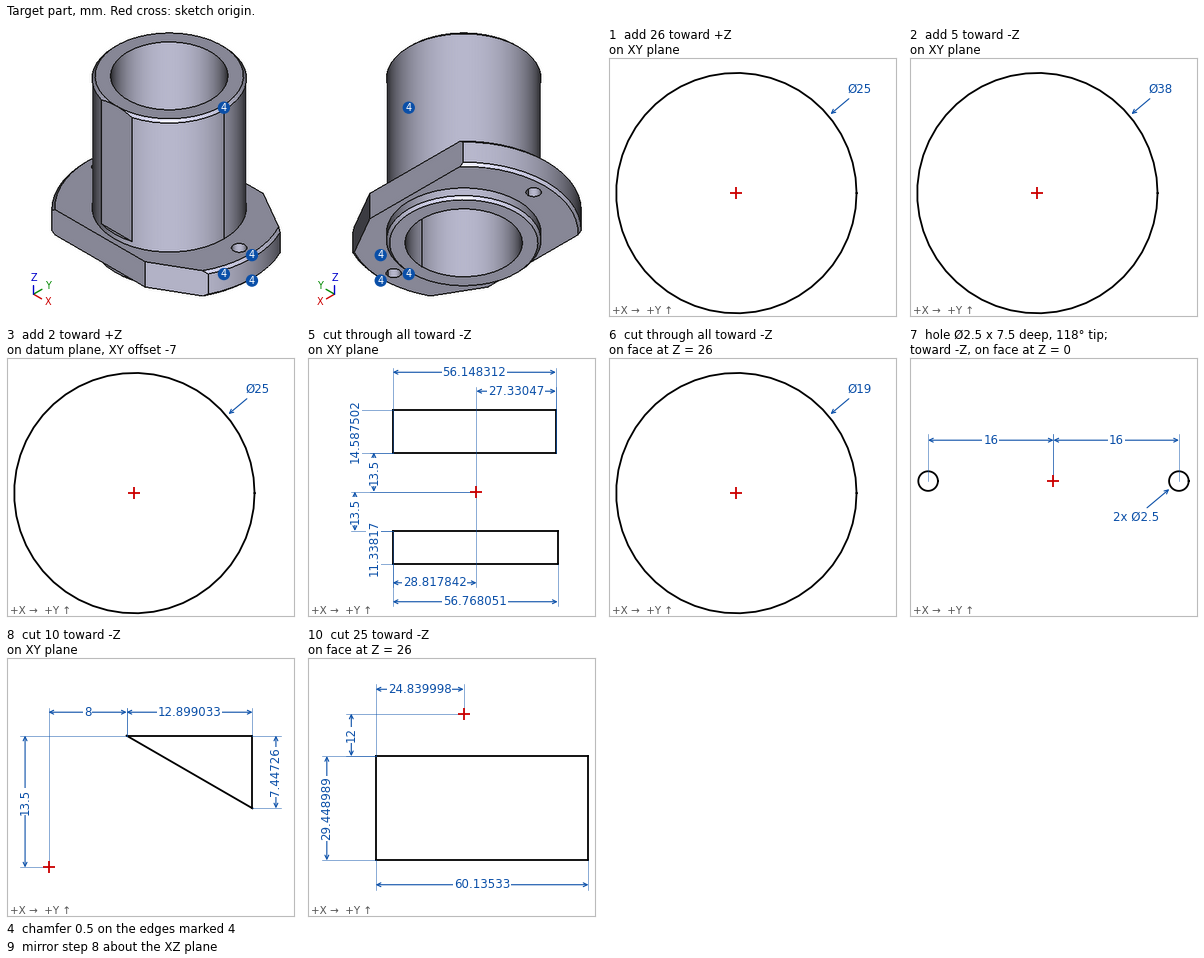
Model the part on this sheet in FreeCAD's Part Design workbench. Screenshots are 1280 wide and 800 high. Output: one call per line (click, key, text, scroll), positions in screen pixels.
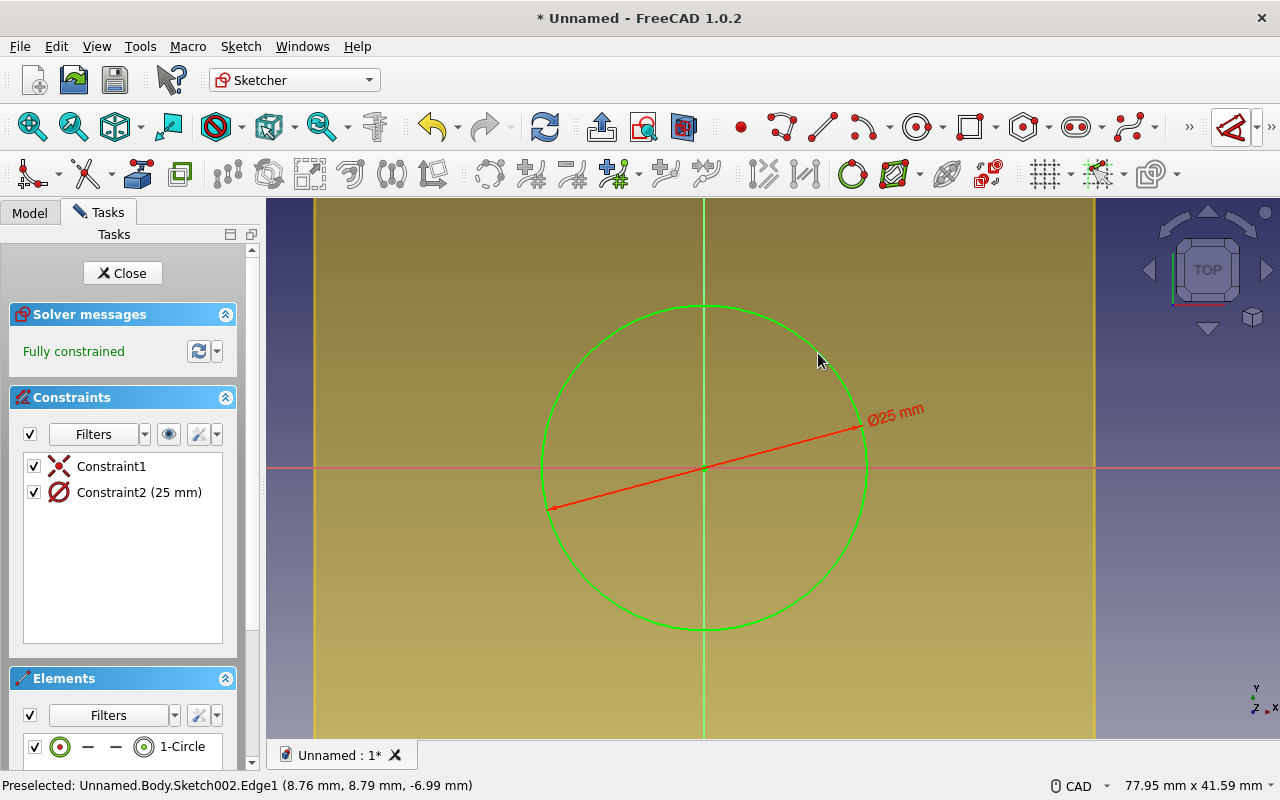
click(123, 273)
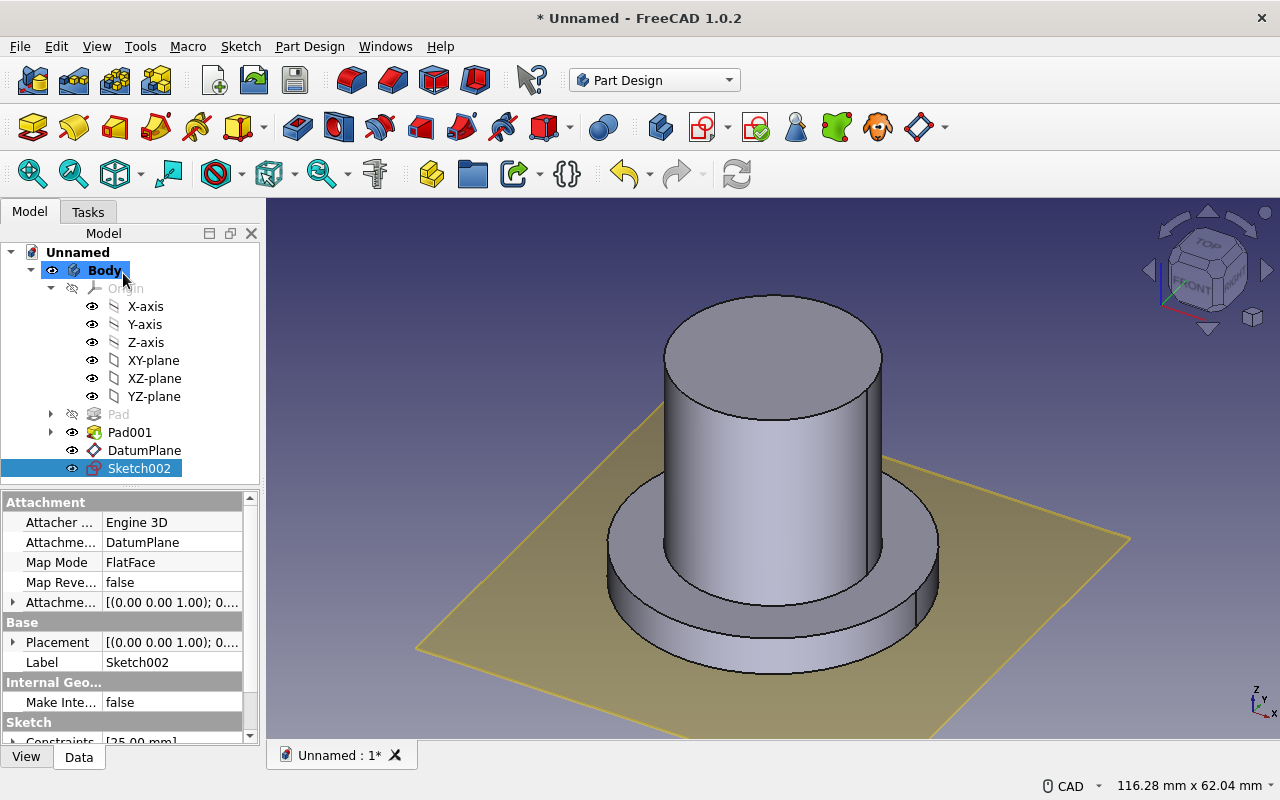
click(33, 128)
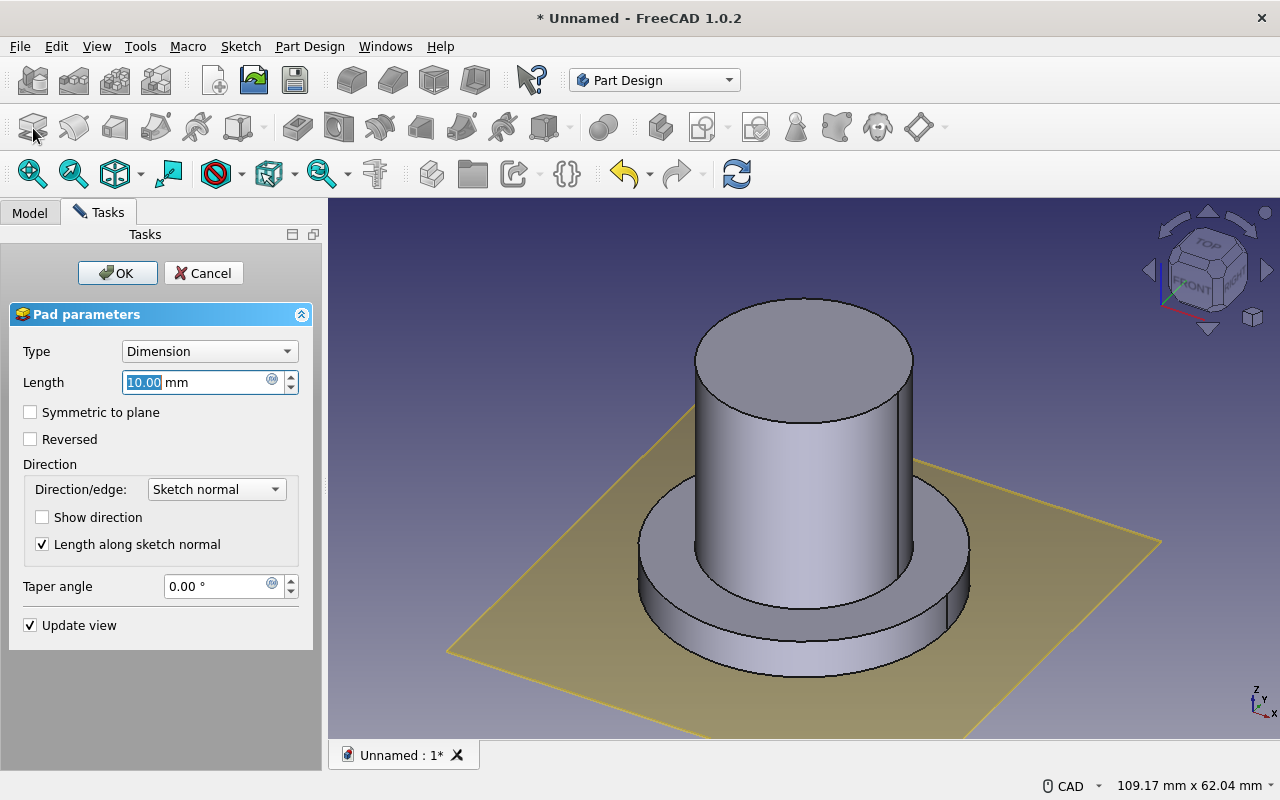
text(2)
key(Tab)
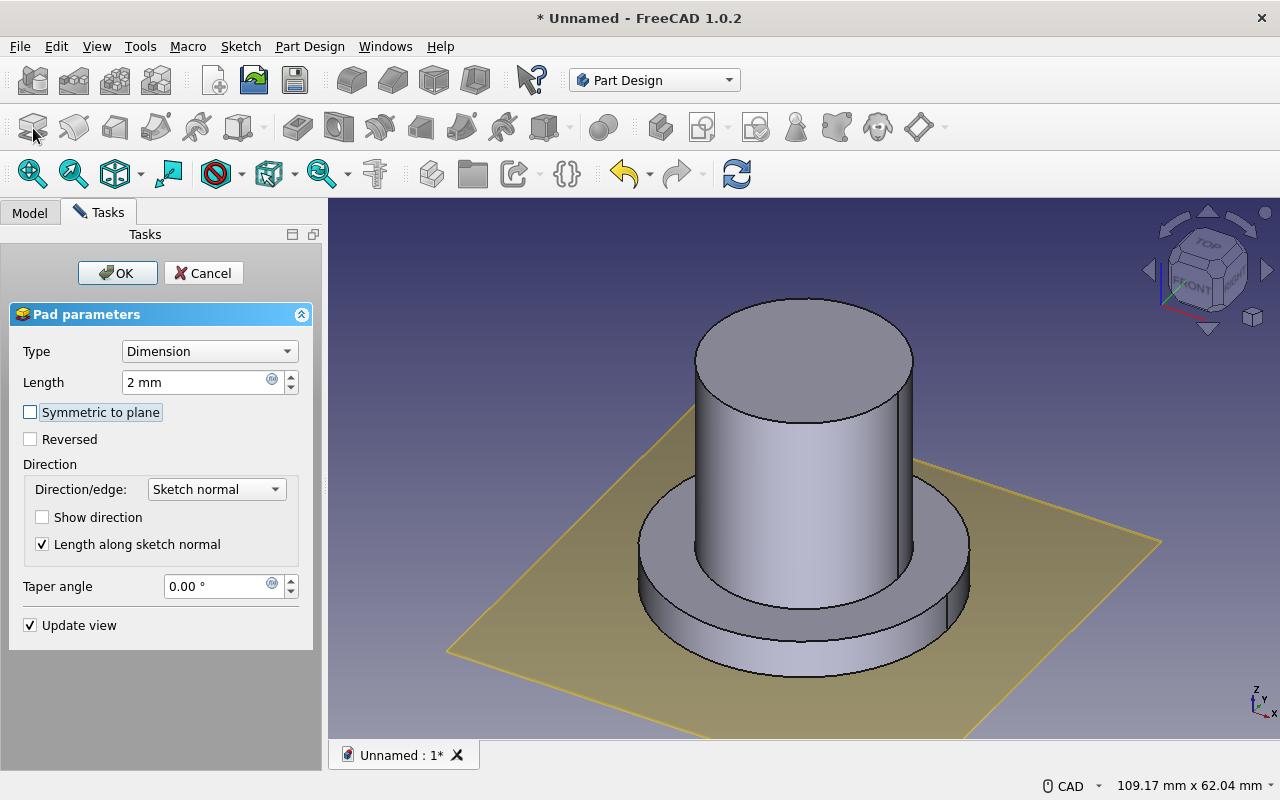
click(118, 273)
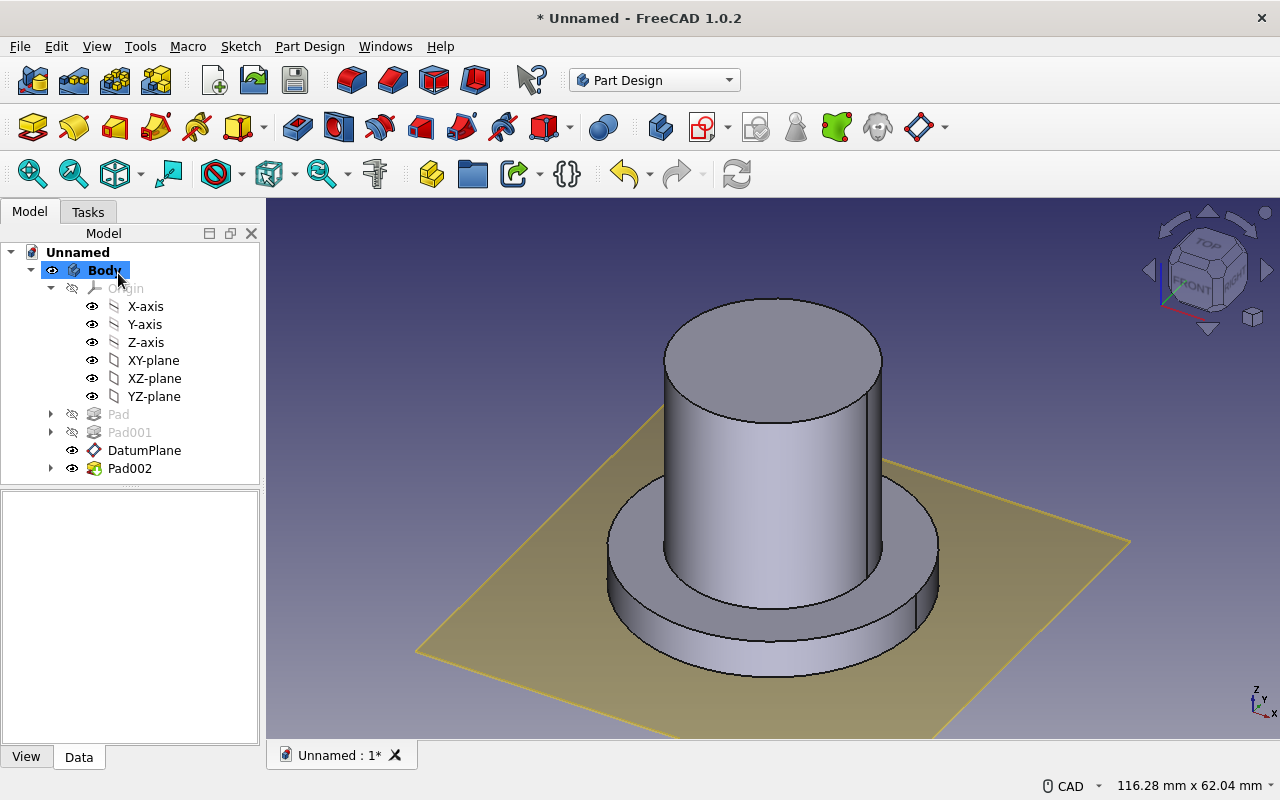
click(117, 450)
key(space)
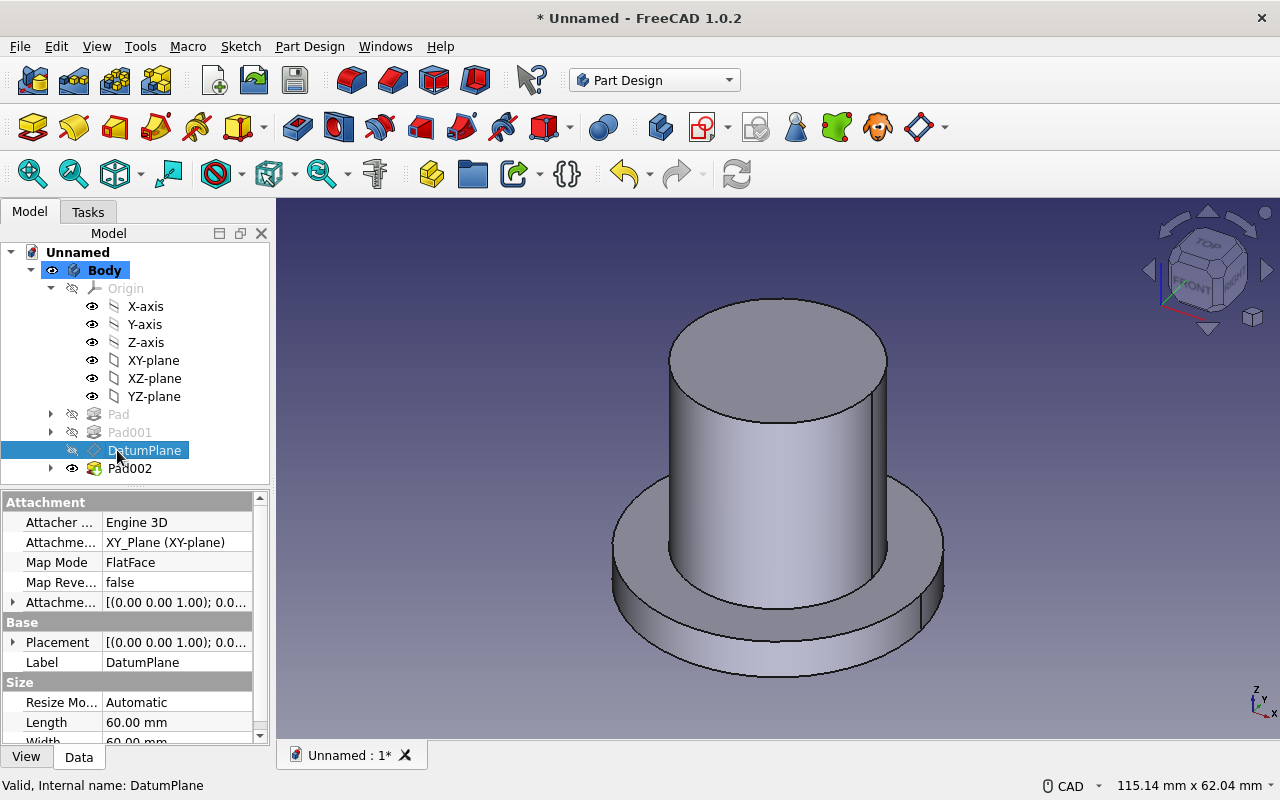
click(670, 366)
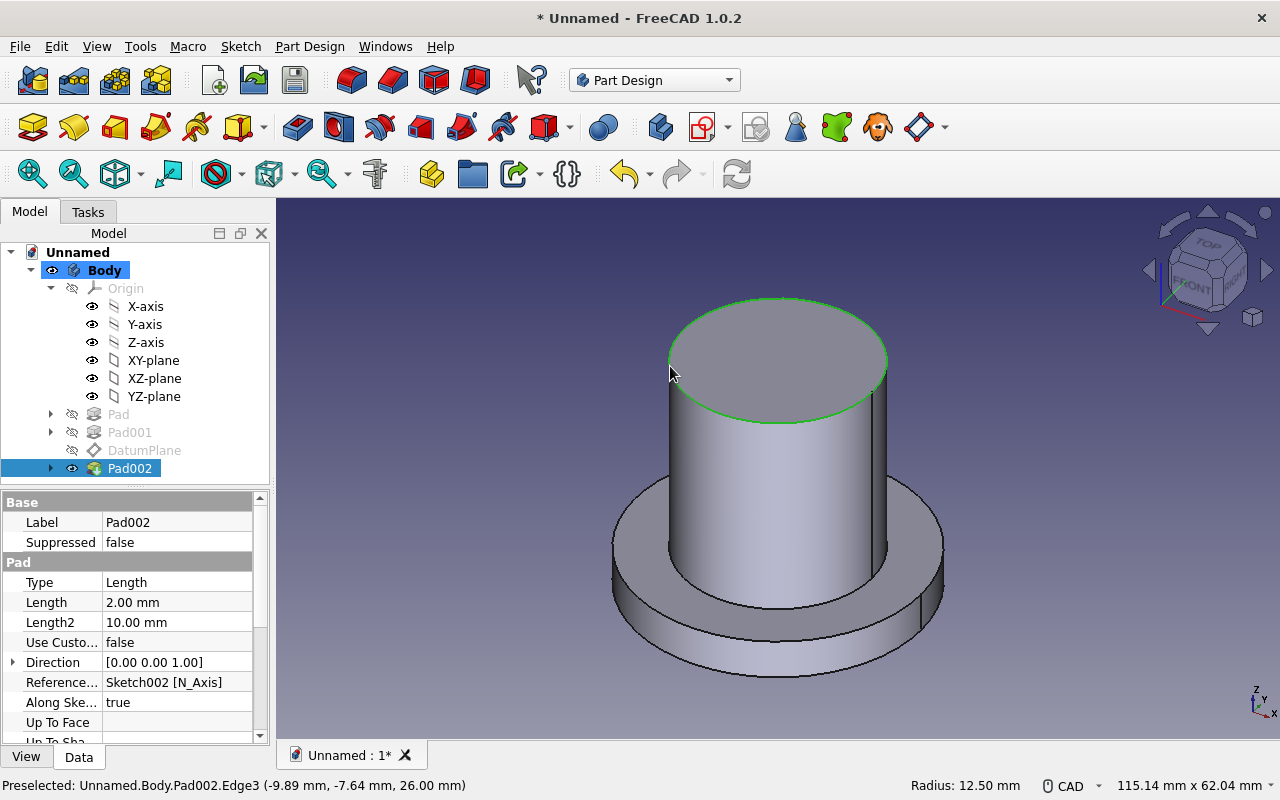
click(613, 556, ctrl)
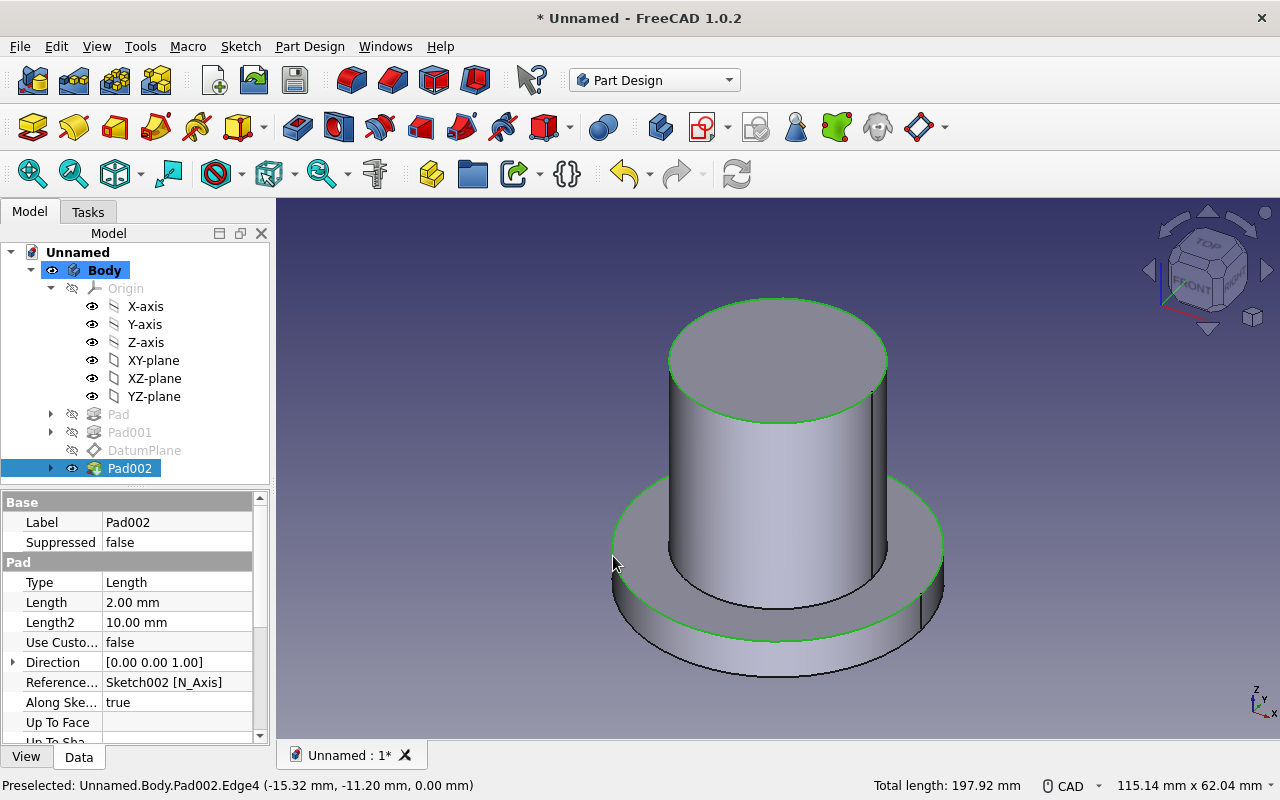
key(0)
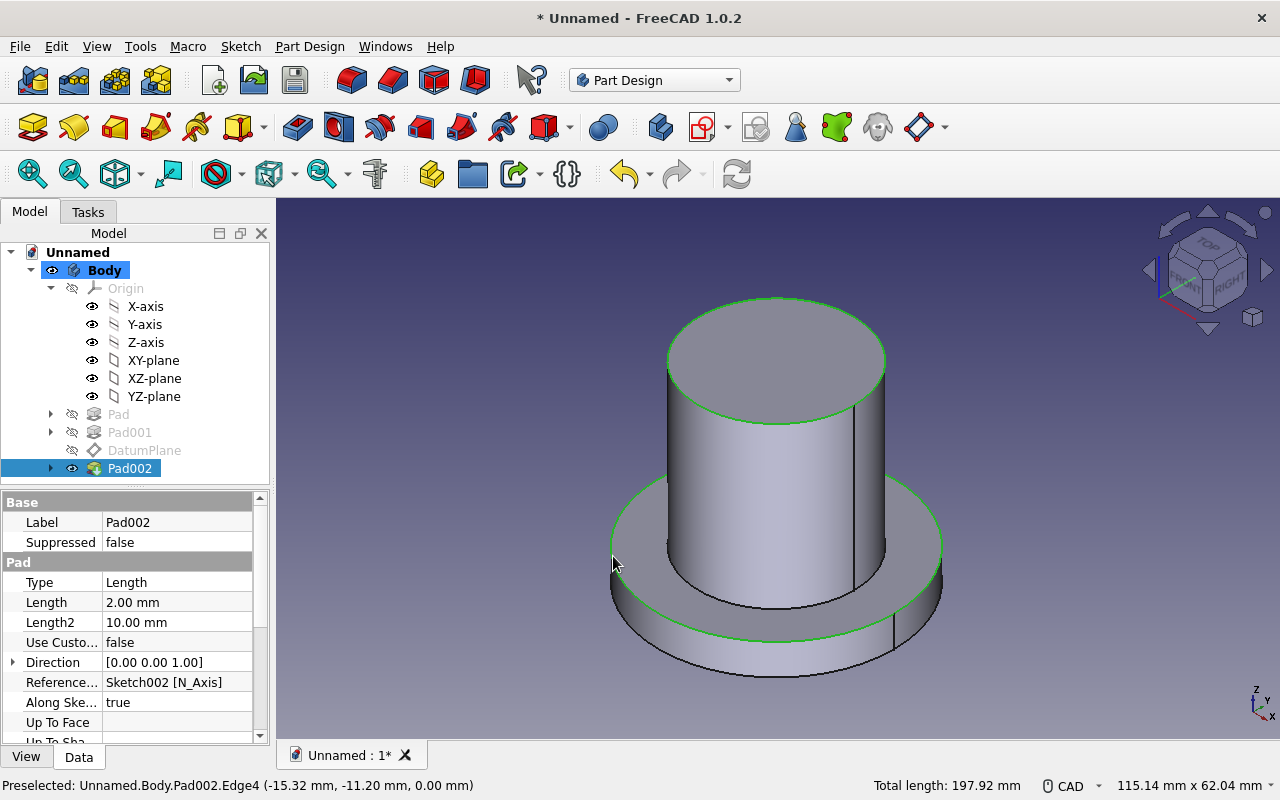
key(2)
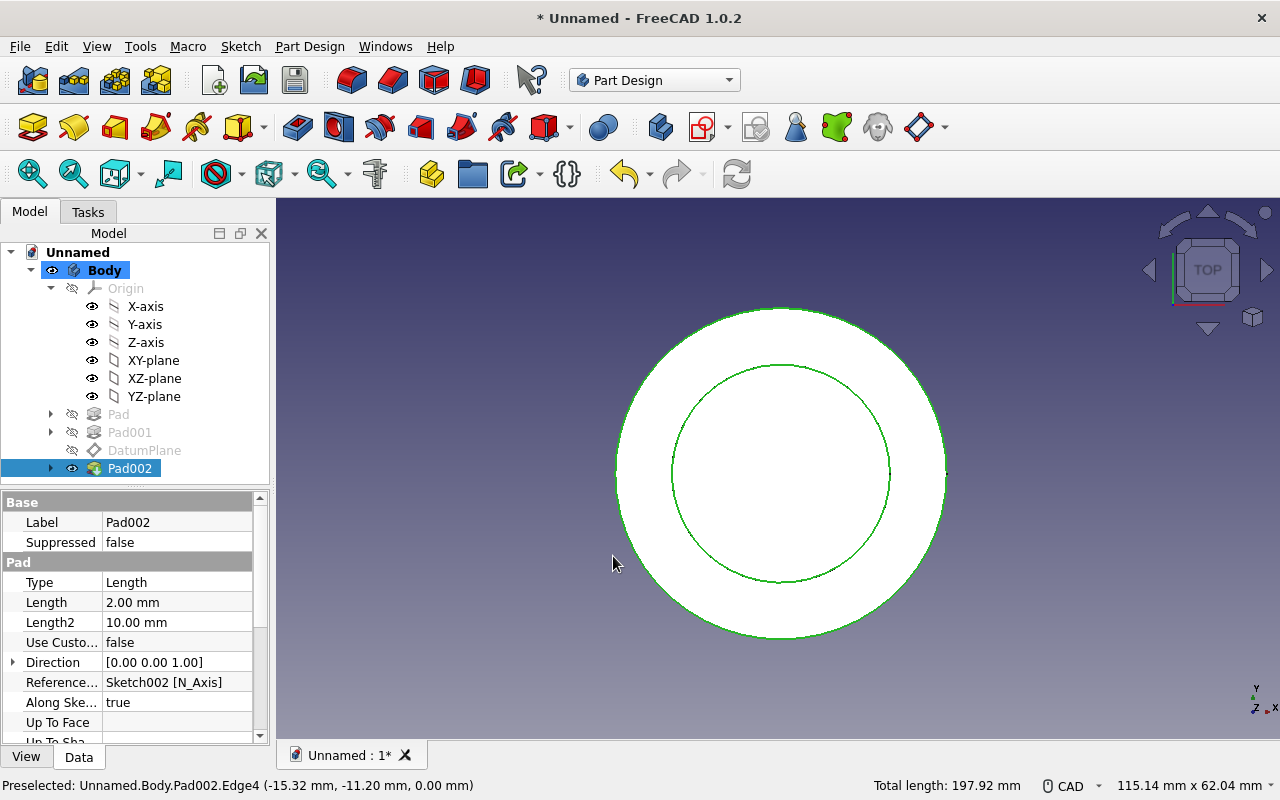
key(1)